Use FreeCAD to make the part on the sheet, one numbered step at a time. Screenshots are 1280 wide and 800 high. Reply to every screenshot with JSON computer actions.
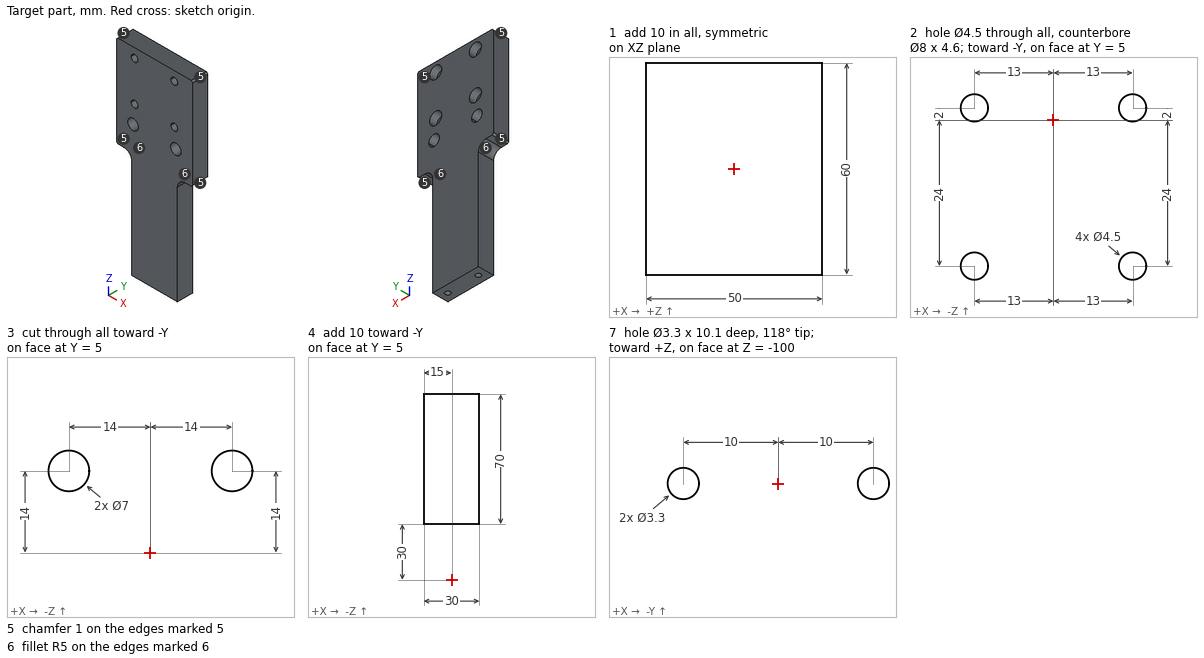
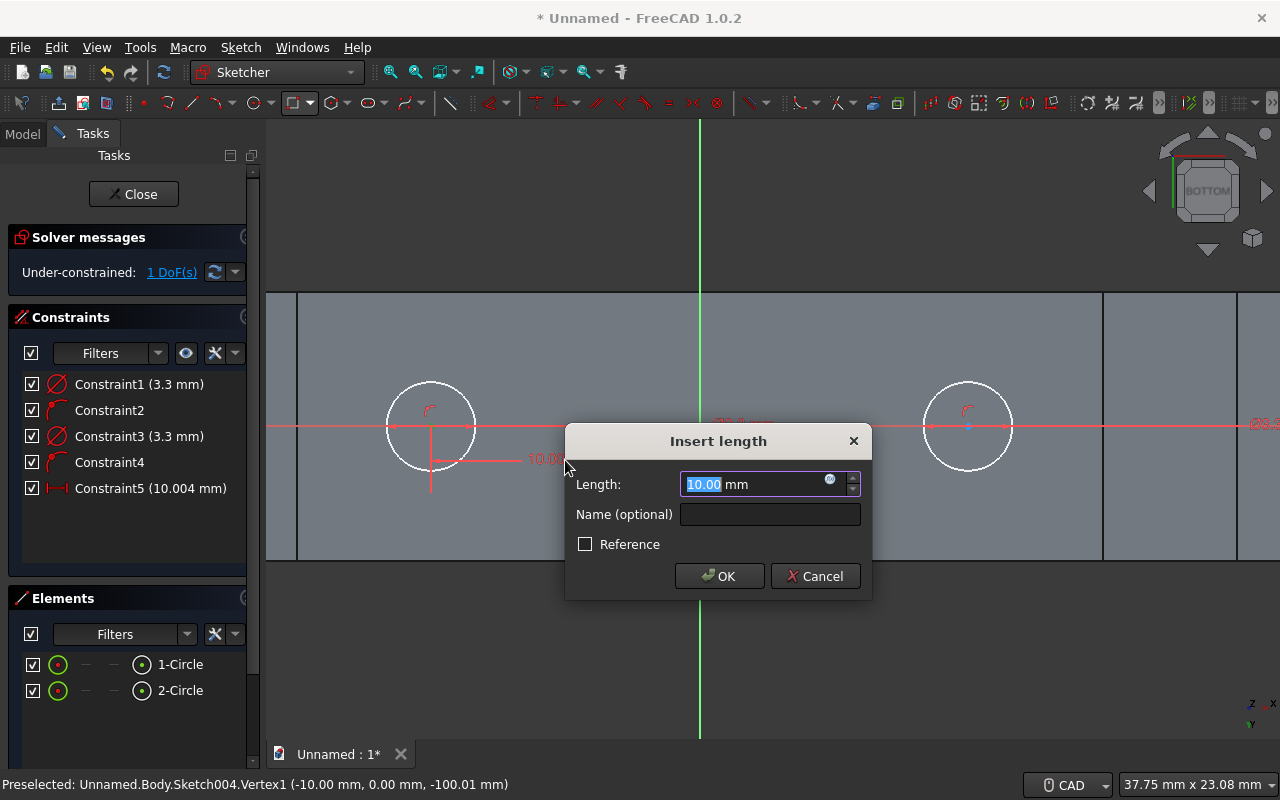
{"action": "type", "text": "10"}
{"action": "key", "text": "Return"}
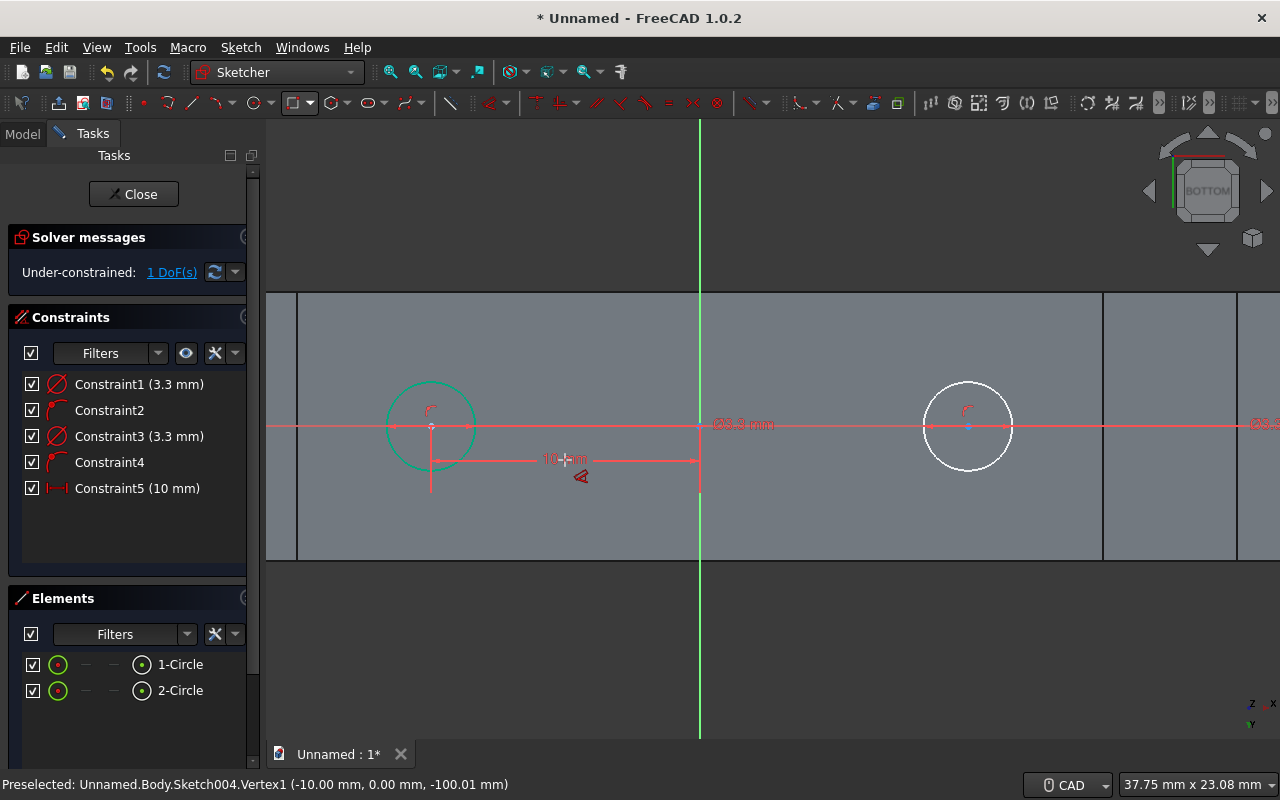
{"action": "left_click", "coordinate": [968, 426]}
{"action": "left_click", "coordinate": [834, 460]}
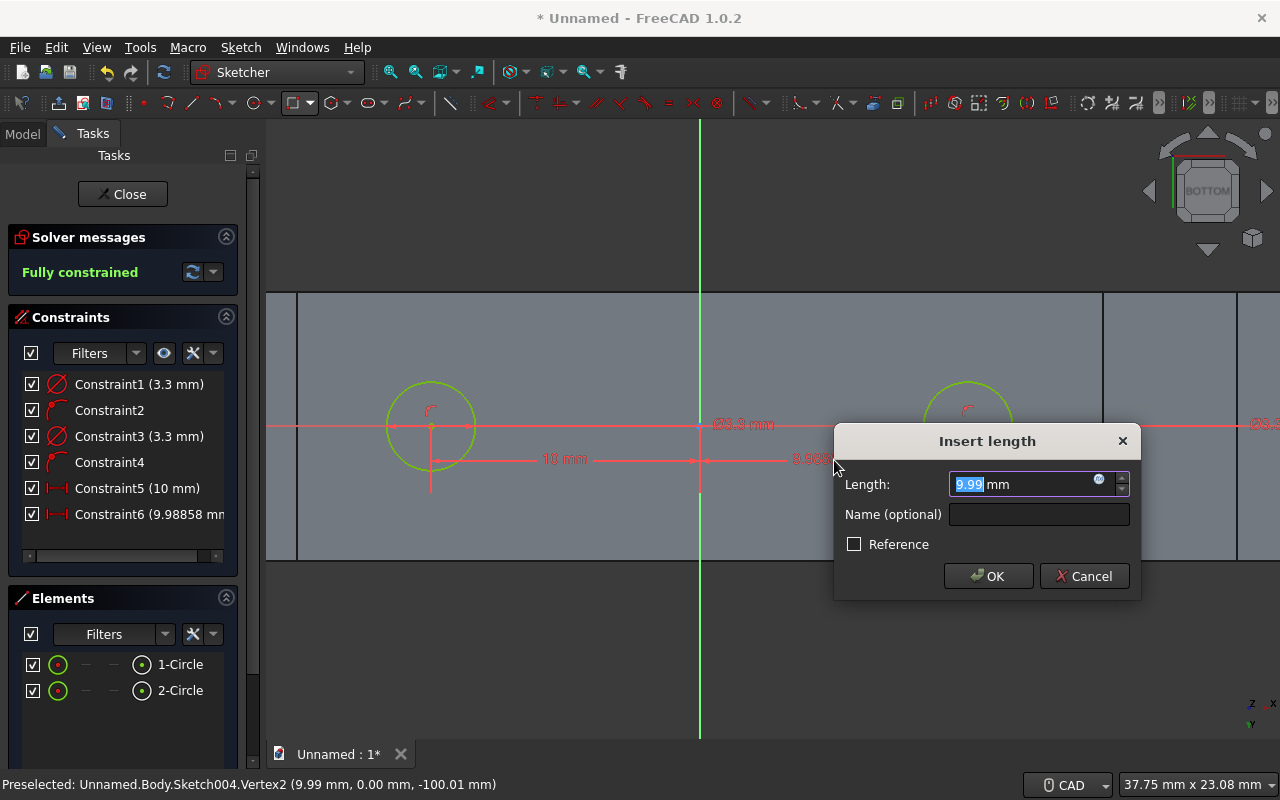
{"action": "type", "text": "10"}
{"action": "key", "text": "Return"}
{"action": "key", "text": "Escape"}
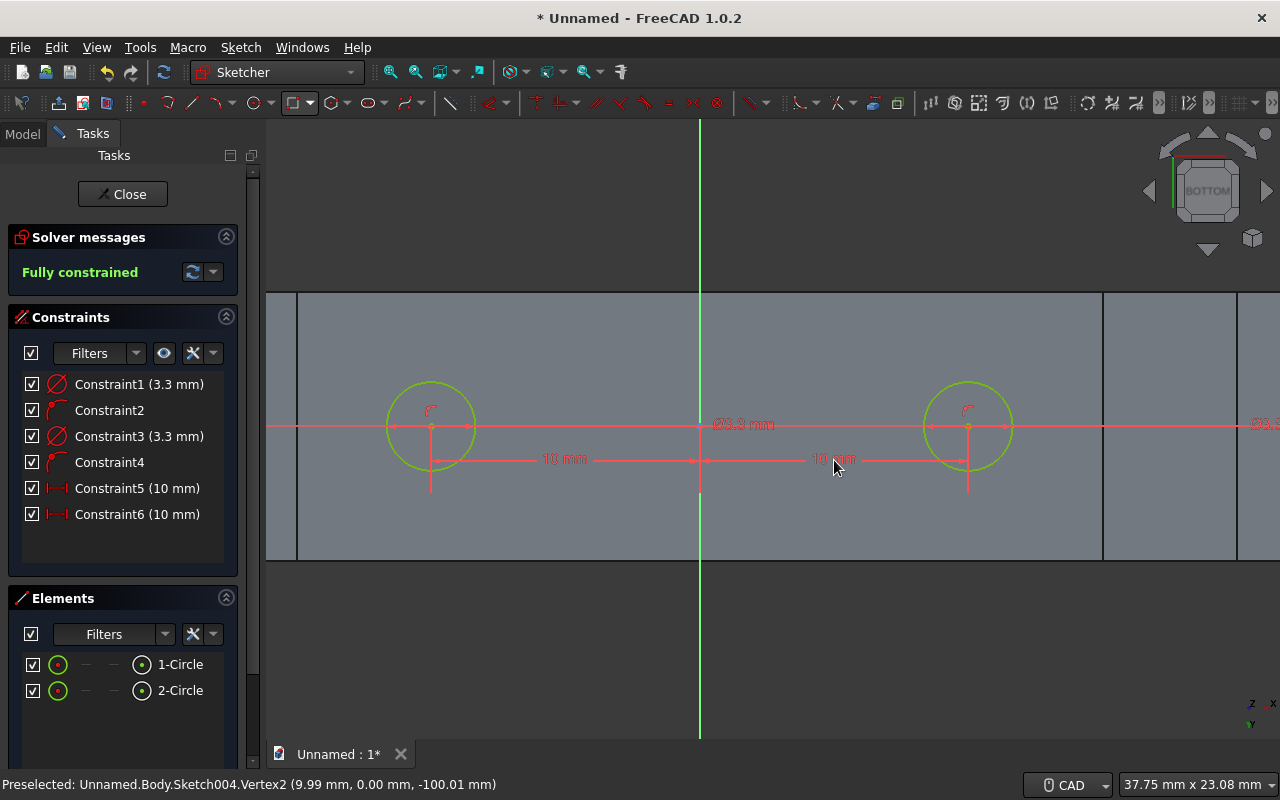
{"action": "left_click", "coordinate": [123, 194]}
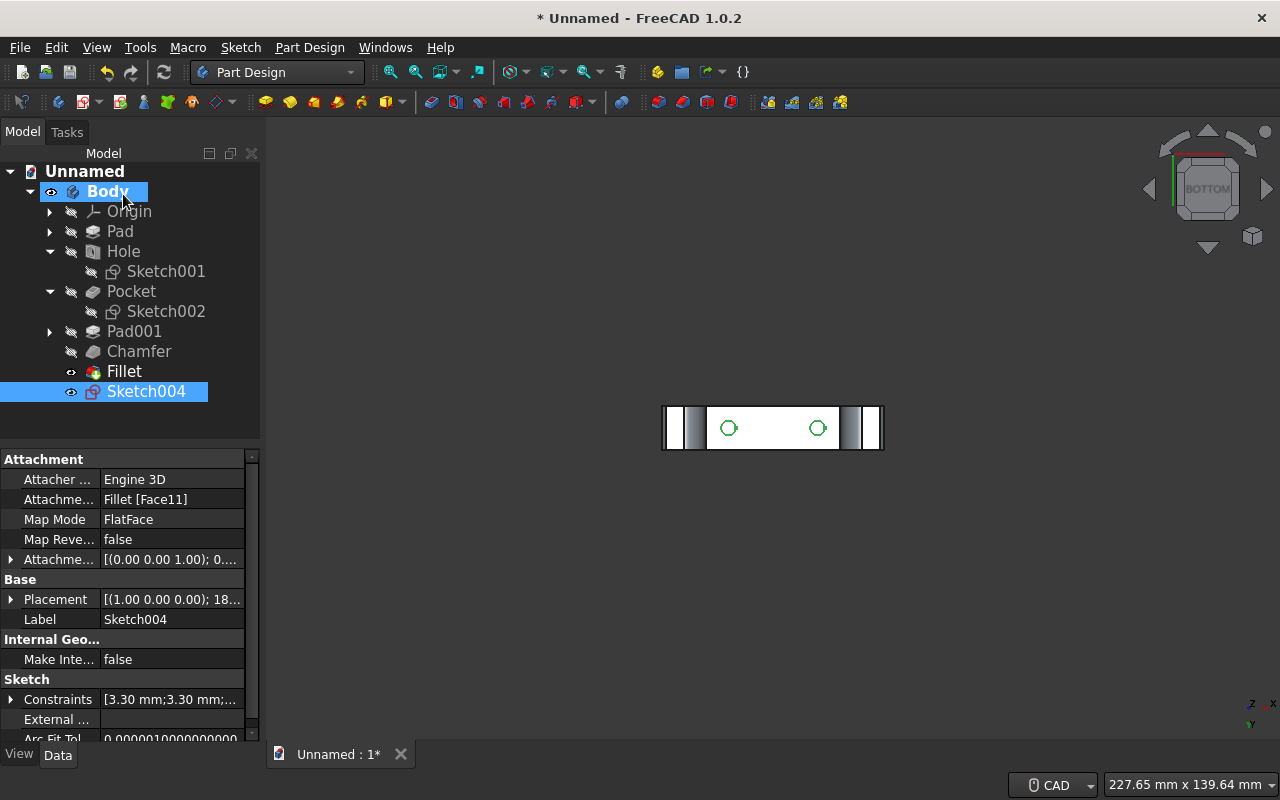
{"action": "left_click", "coordinate": [456, 102]}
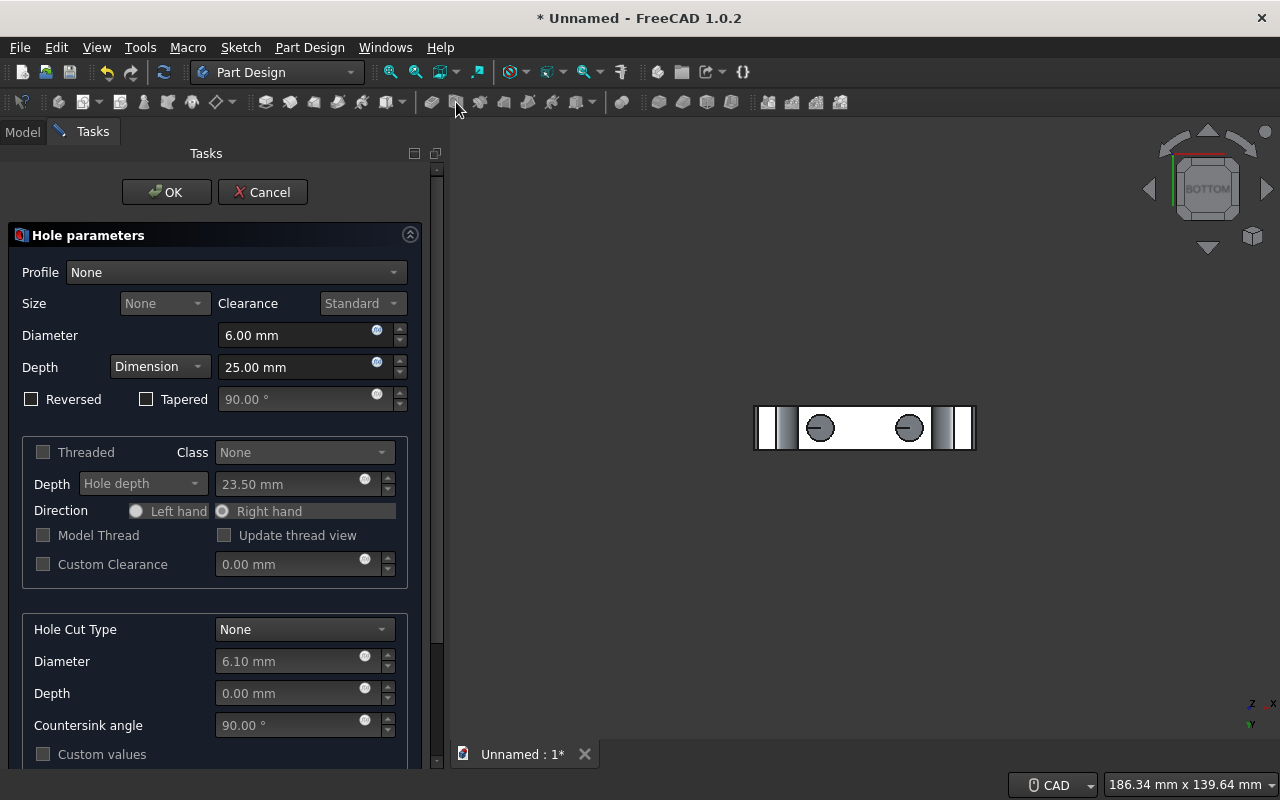
{"action": "triple_click", "coordinate": [305, 335]}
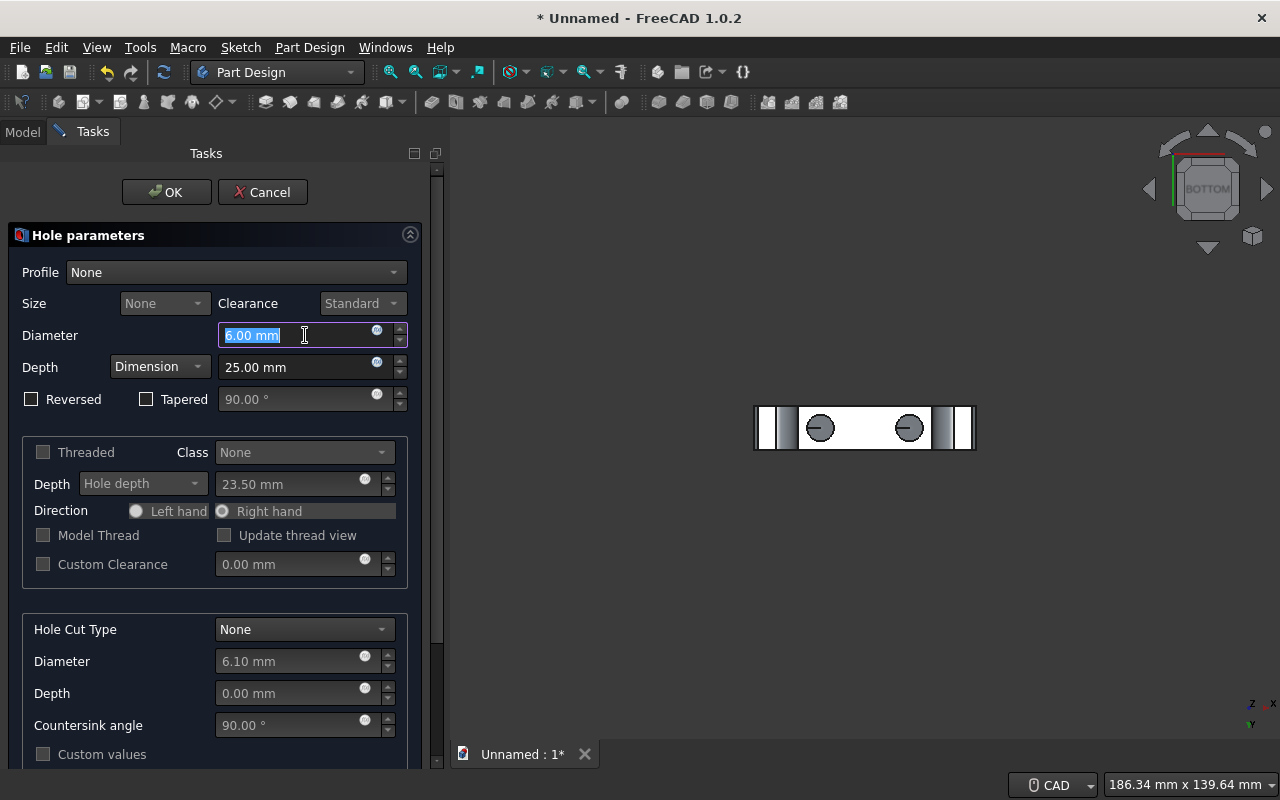
{"action": "type", "text": "3.3"}
{"action": "key", "text": "Tab"}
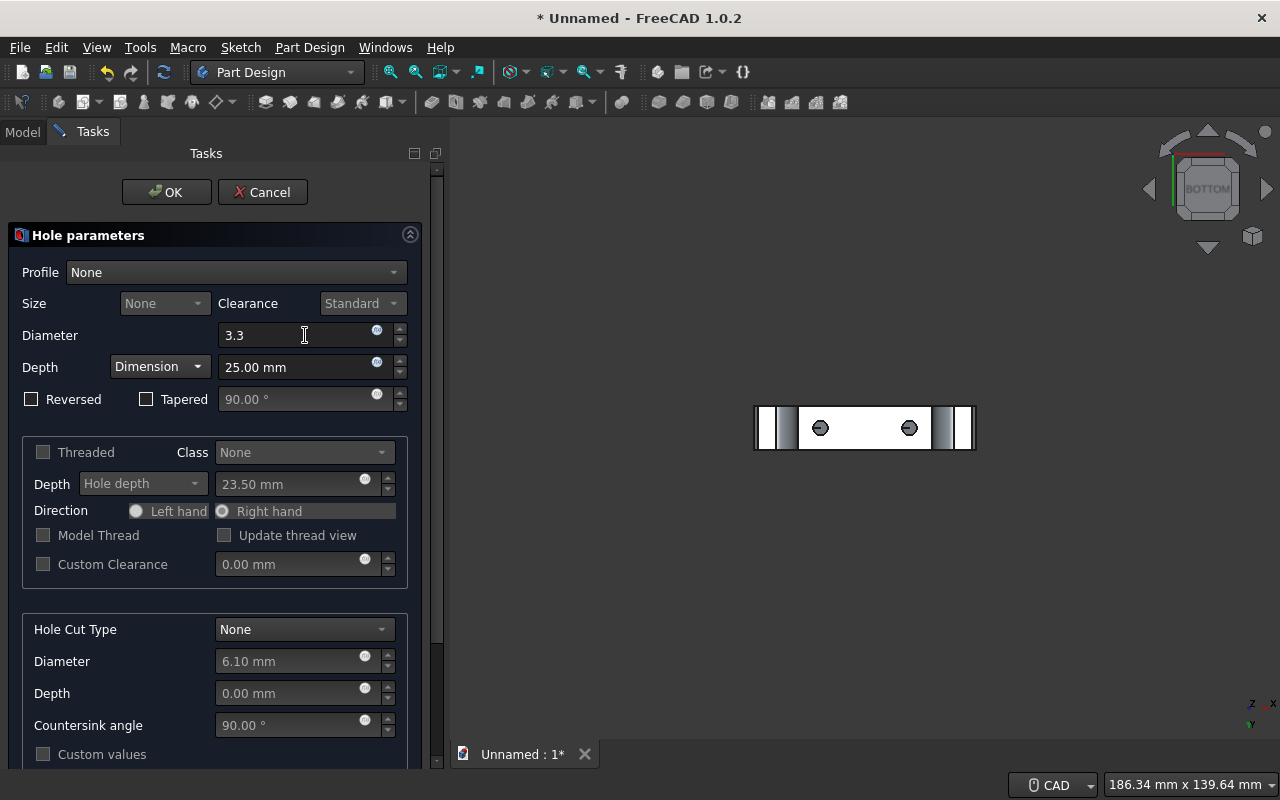
{"action": "triple_click", "coordinate": [305, 367]}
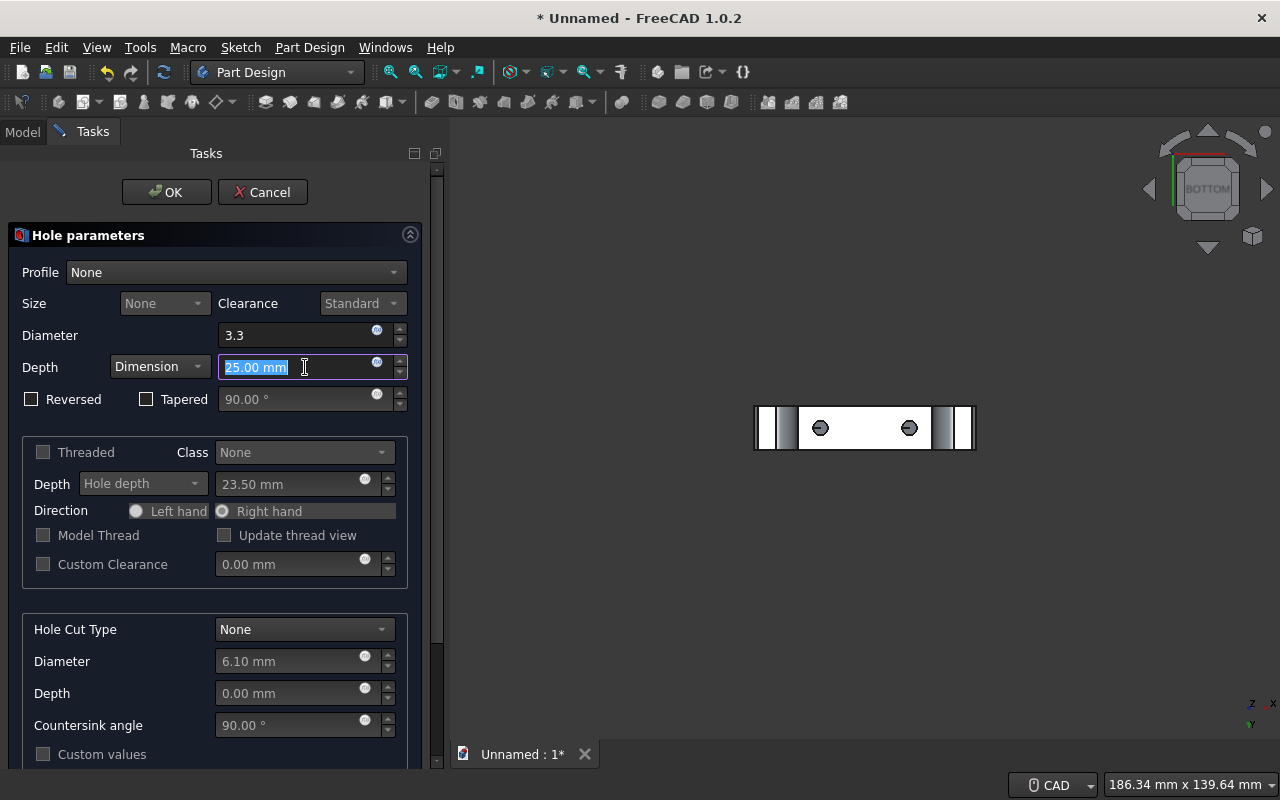
{"action": "type", "text": "10.1"}
{"action": "key", "text": "Tab"}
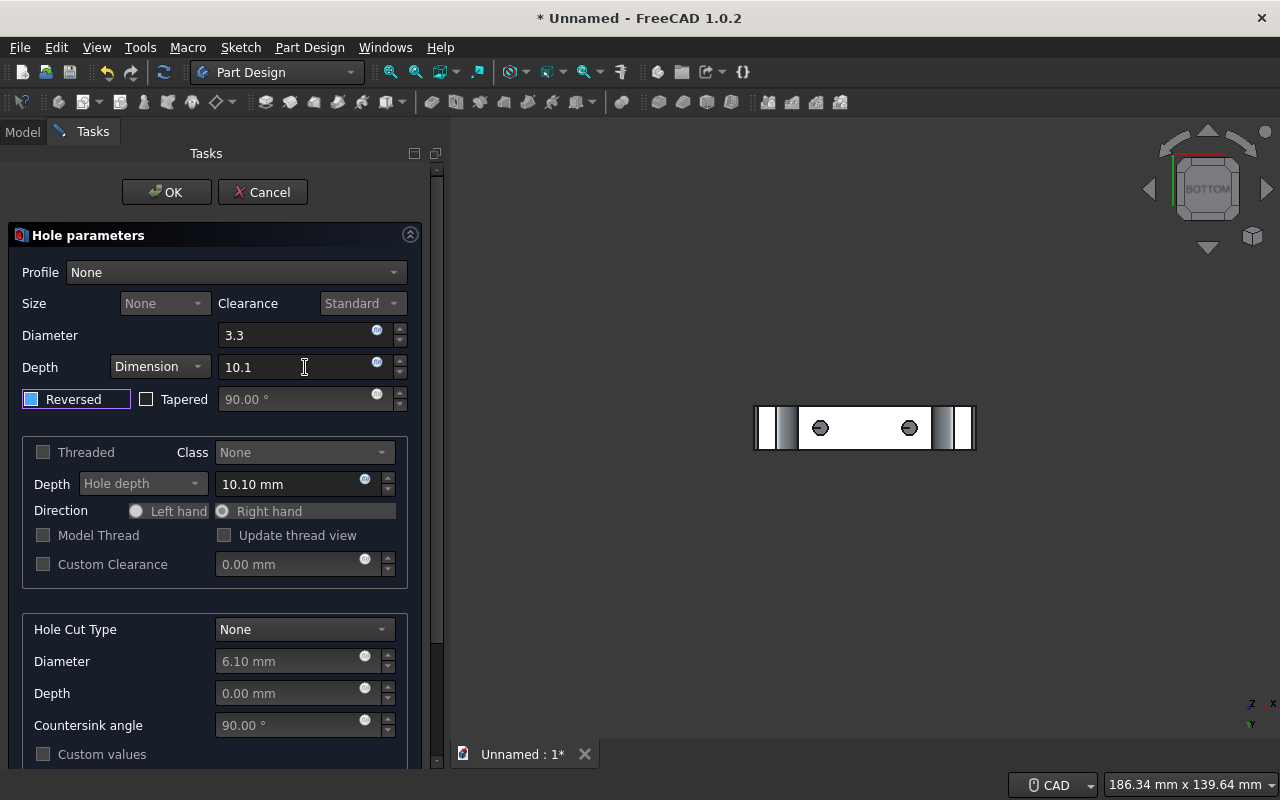
{"action": "left_click", "coordinate": [167, 192]}